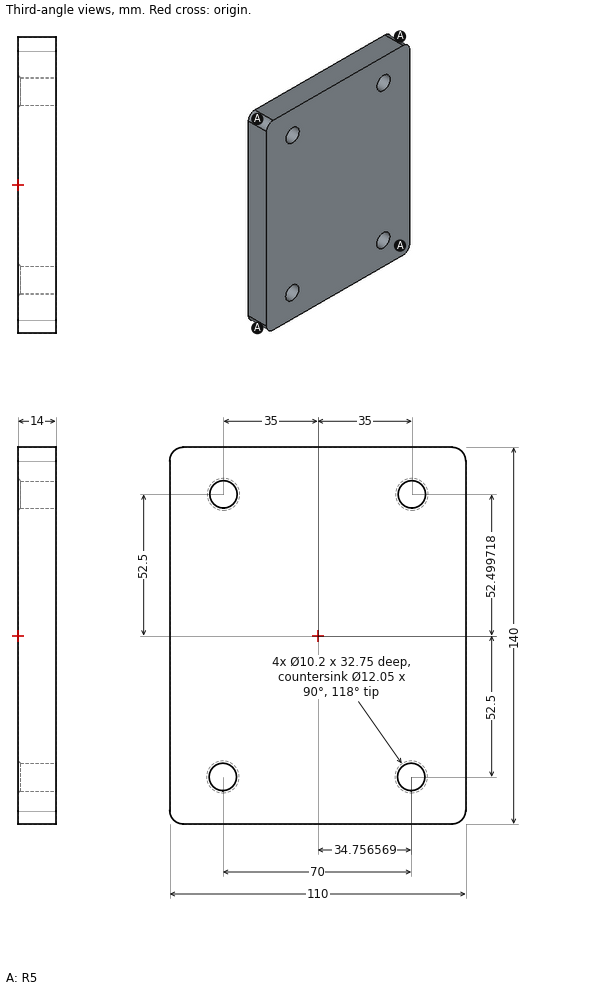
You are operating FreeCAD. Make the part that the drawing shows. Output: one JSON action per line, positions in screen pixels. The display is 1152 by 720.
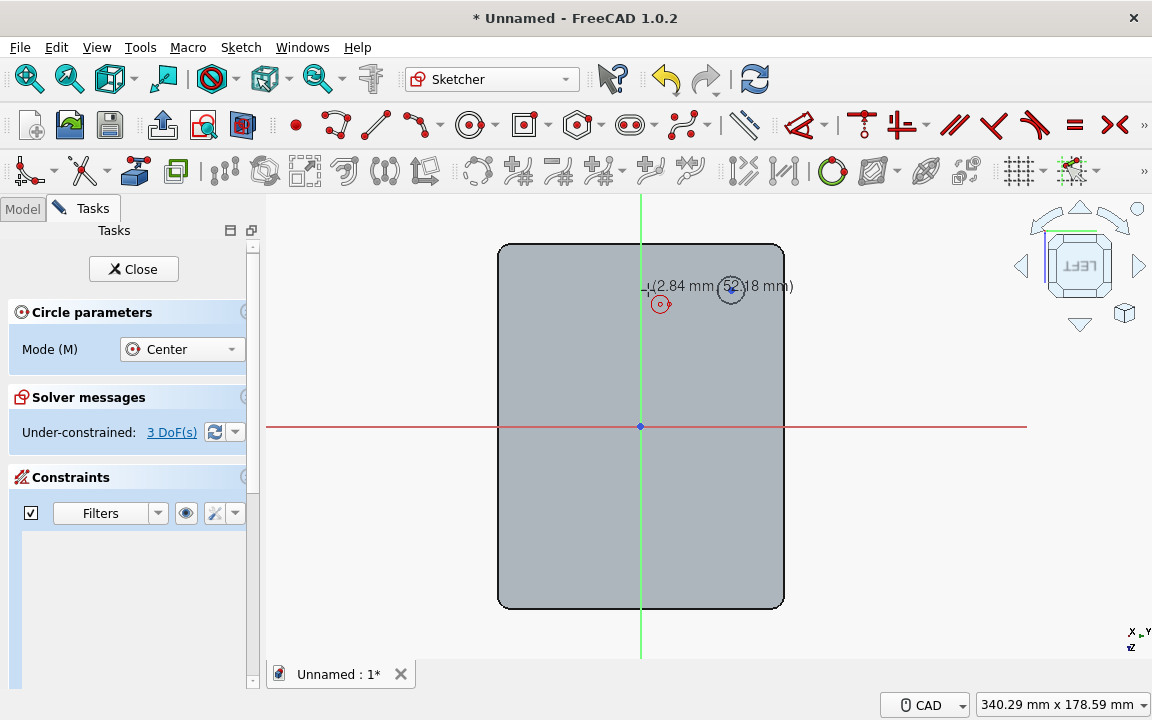
{"action": "scroll", "coordinate": [732, 563], "scroll_direction": "up", "scroll_amount": 3}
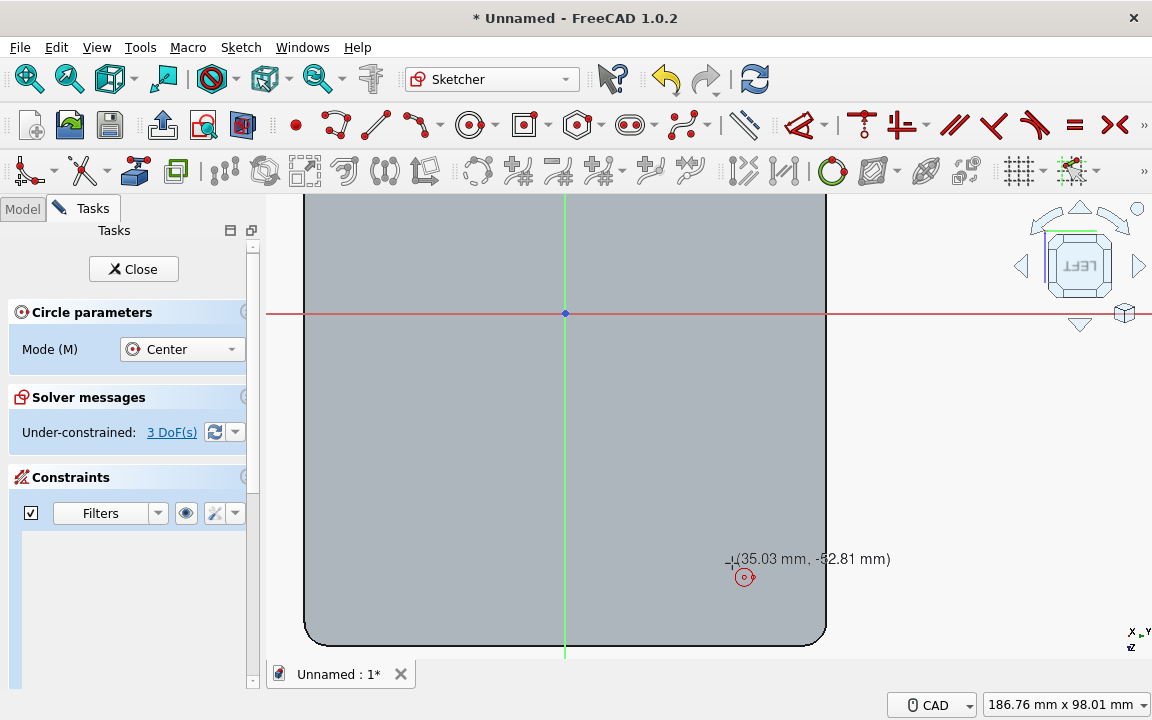
{"action": "left_click", "coordinate": [731, 563]}
{"action": "left_click", "coordinate": [749, 546]}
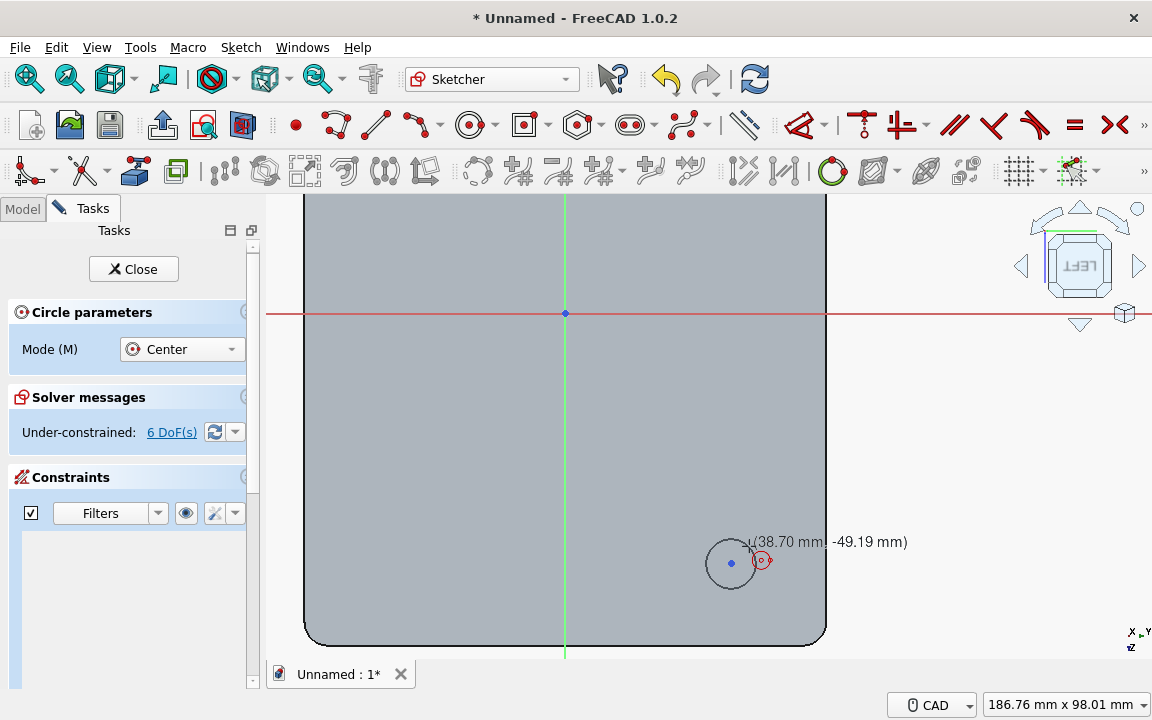
{"action": "left_click", "coordinate": [399, 563]}
{"action": "left_click", "coordinate": [416, 546]}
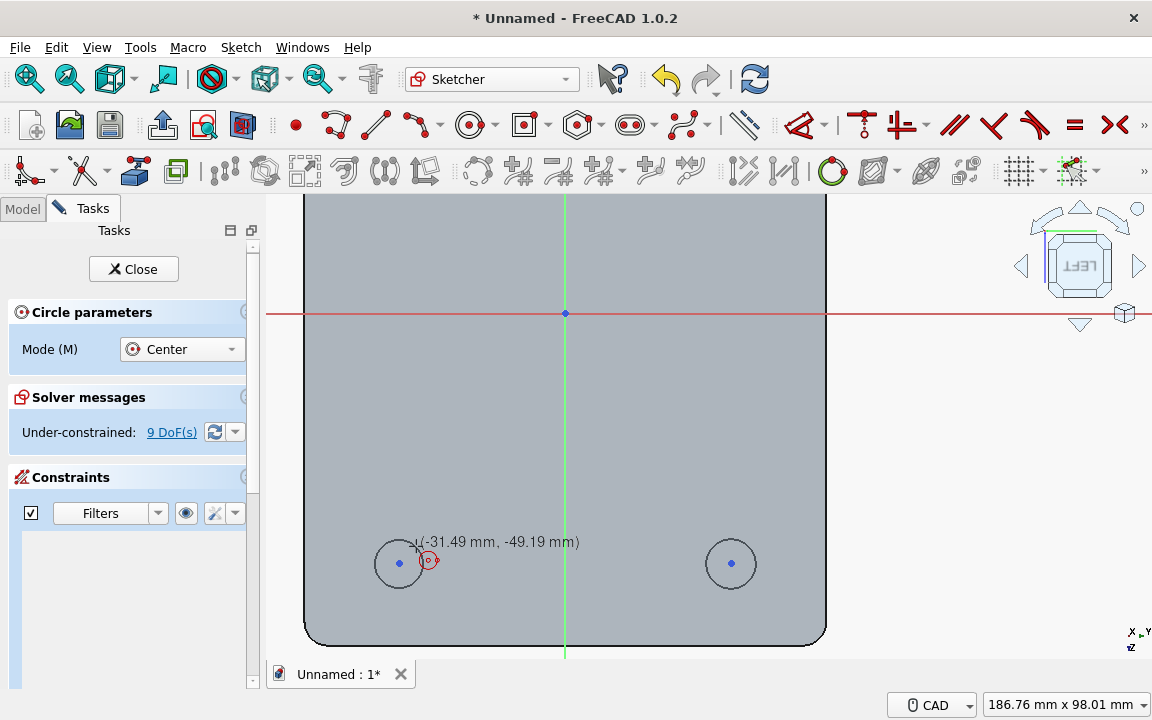
{"action": "scroll", "coordinate": [733, 564], "scroll_direction": "down", "scroll_amount": 3}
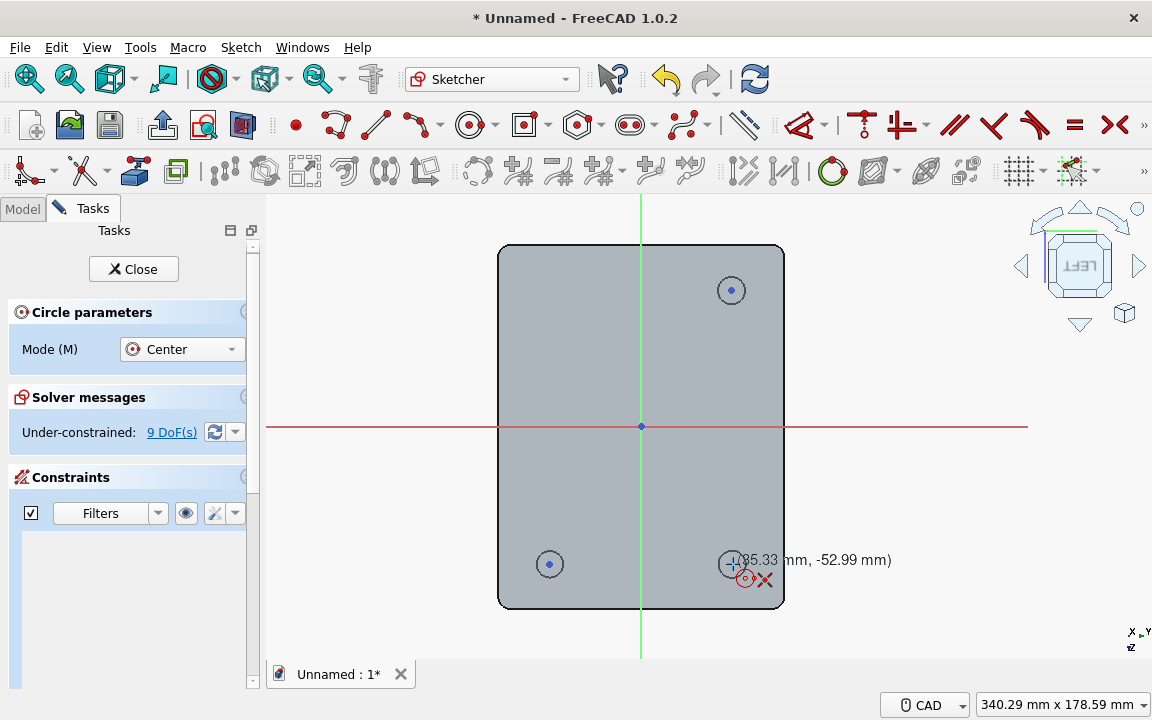
{"action": "scroll", "coordinate": [549, 290], "scroll_direction": "up", "scroll_amount": 3}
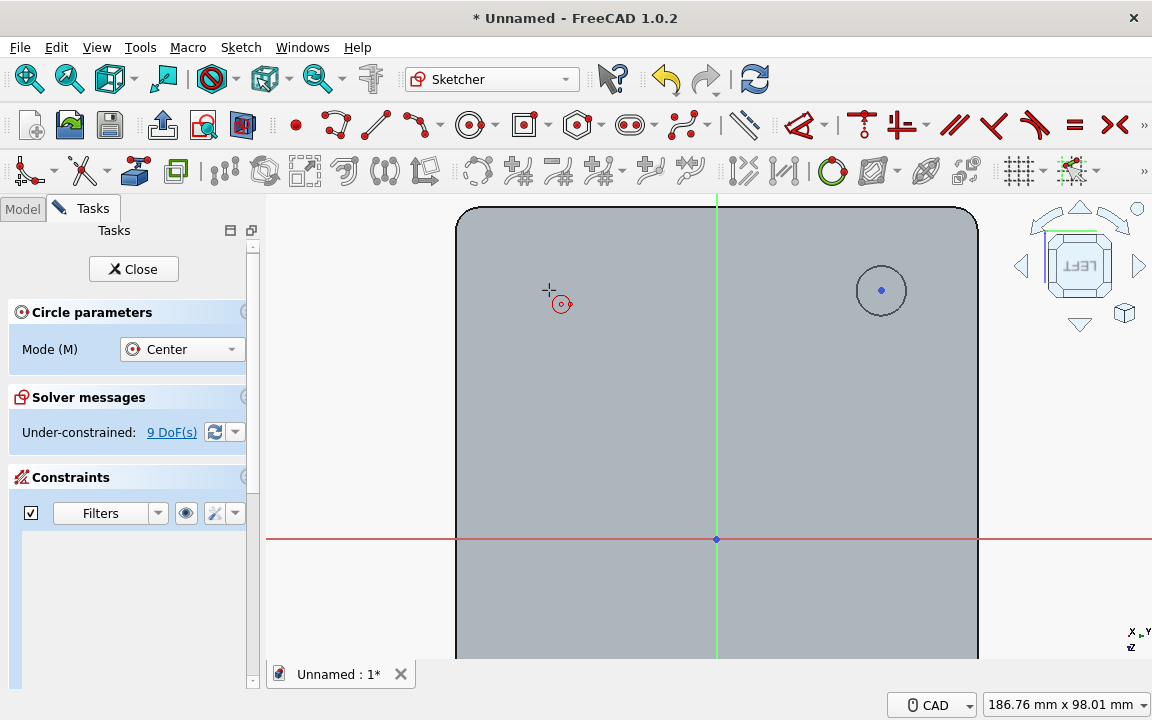
{"action": "left_click", "coordinate": [550, 290]}
{"action": "left_click", "coordinate": [567, 273]}
{"action": "key", "text": "Escape"}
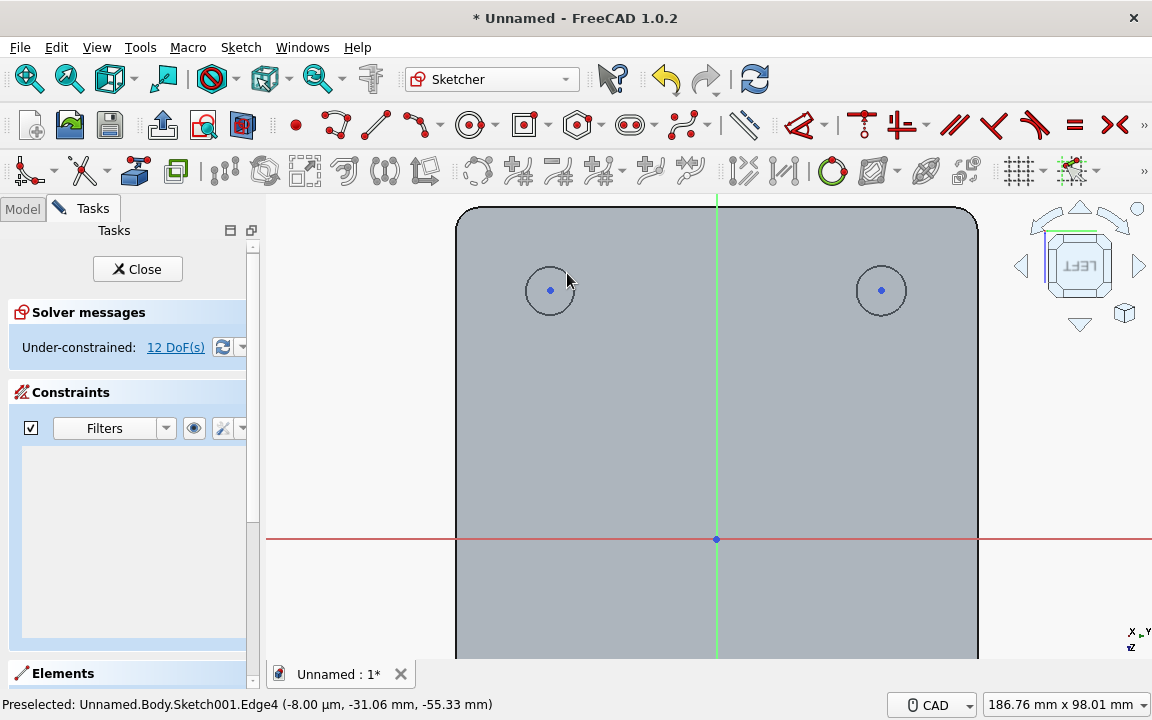
{"action": "left_click", "coordinate": [899, 273]}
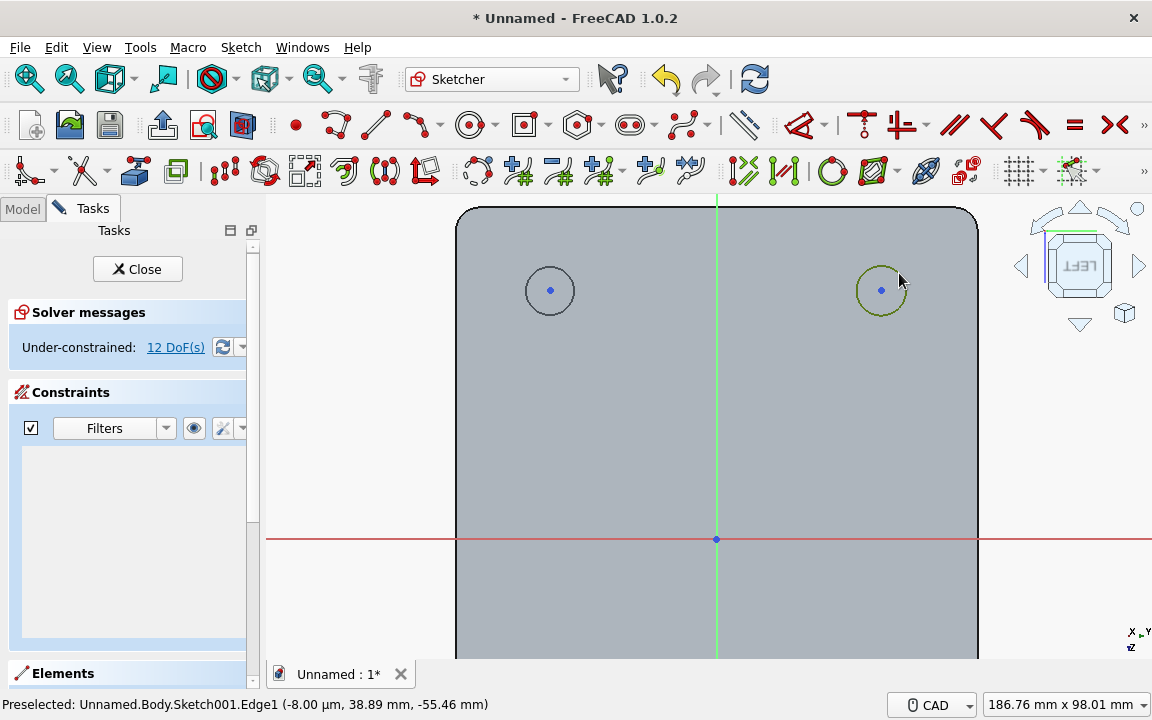
{"action": "scroll", "coordinate": [548, 289], "scroll_direction": "down", "scroll_amount": 3}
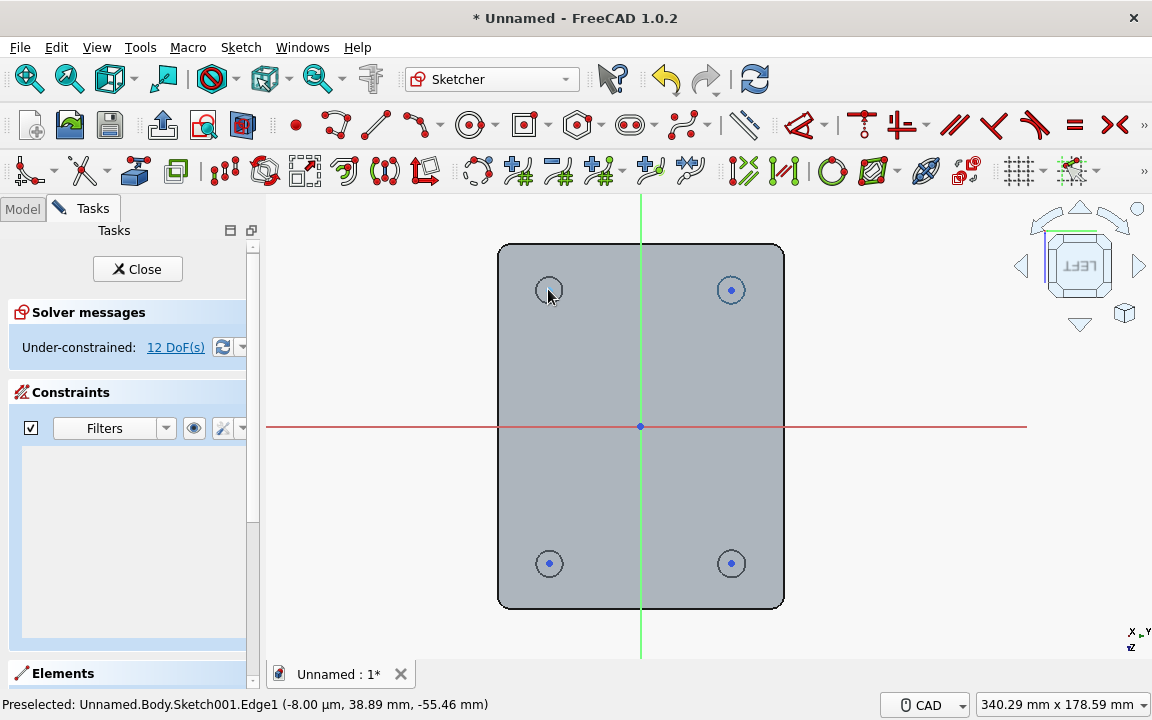
{"action": "left_click", "coordinate": [741, 554]}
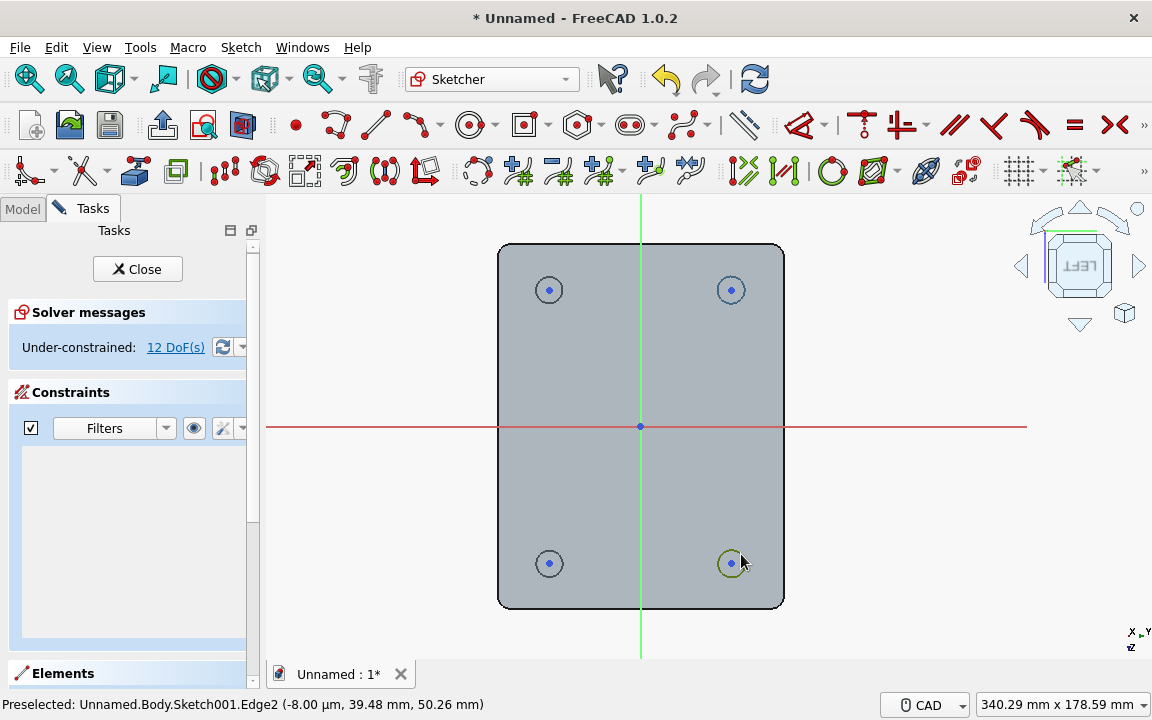
{"action": "left_click", "coordinate": [559, 555]}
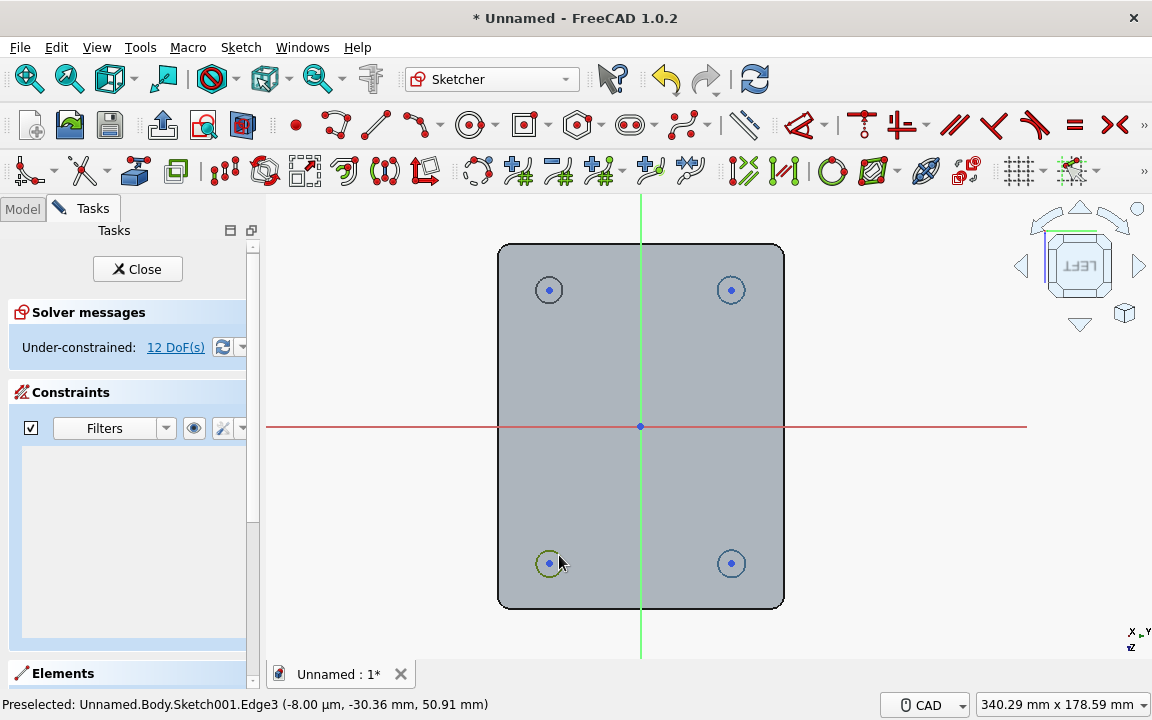
{"action": "left_click", "coordinate": [559, 281]}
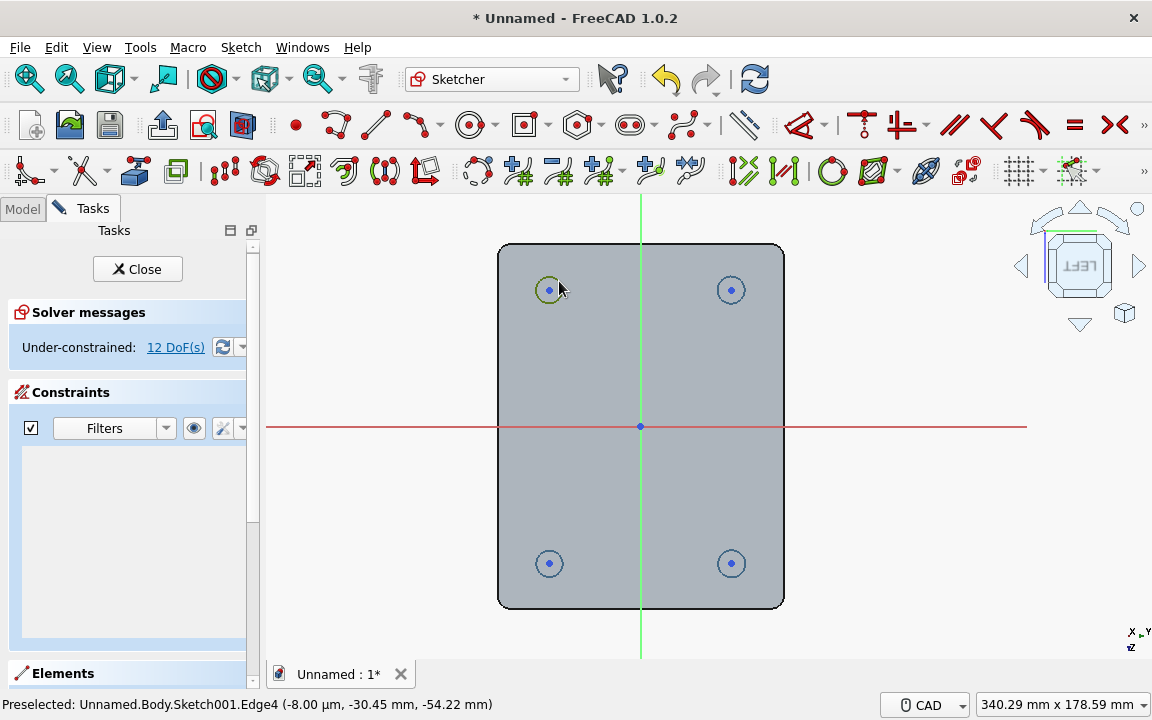
{"action": "left_click", "coordinate": [1076, 126]}